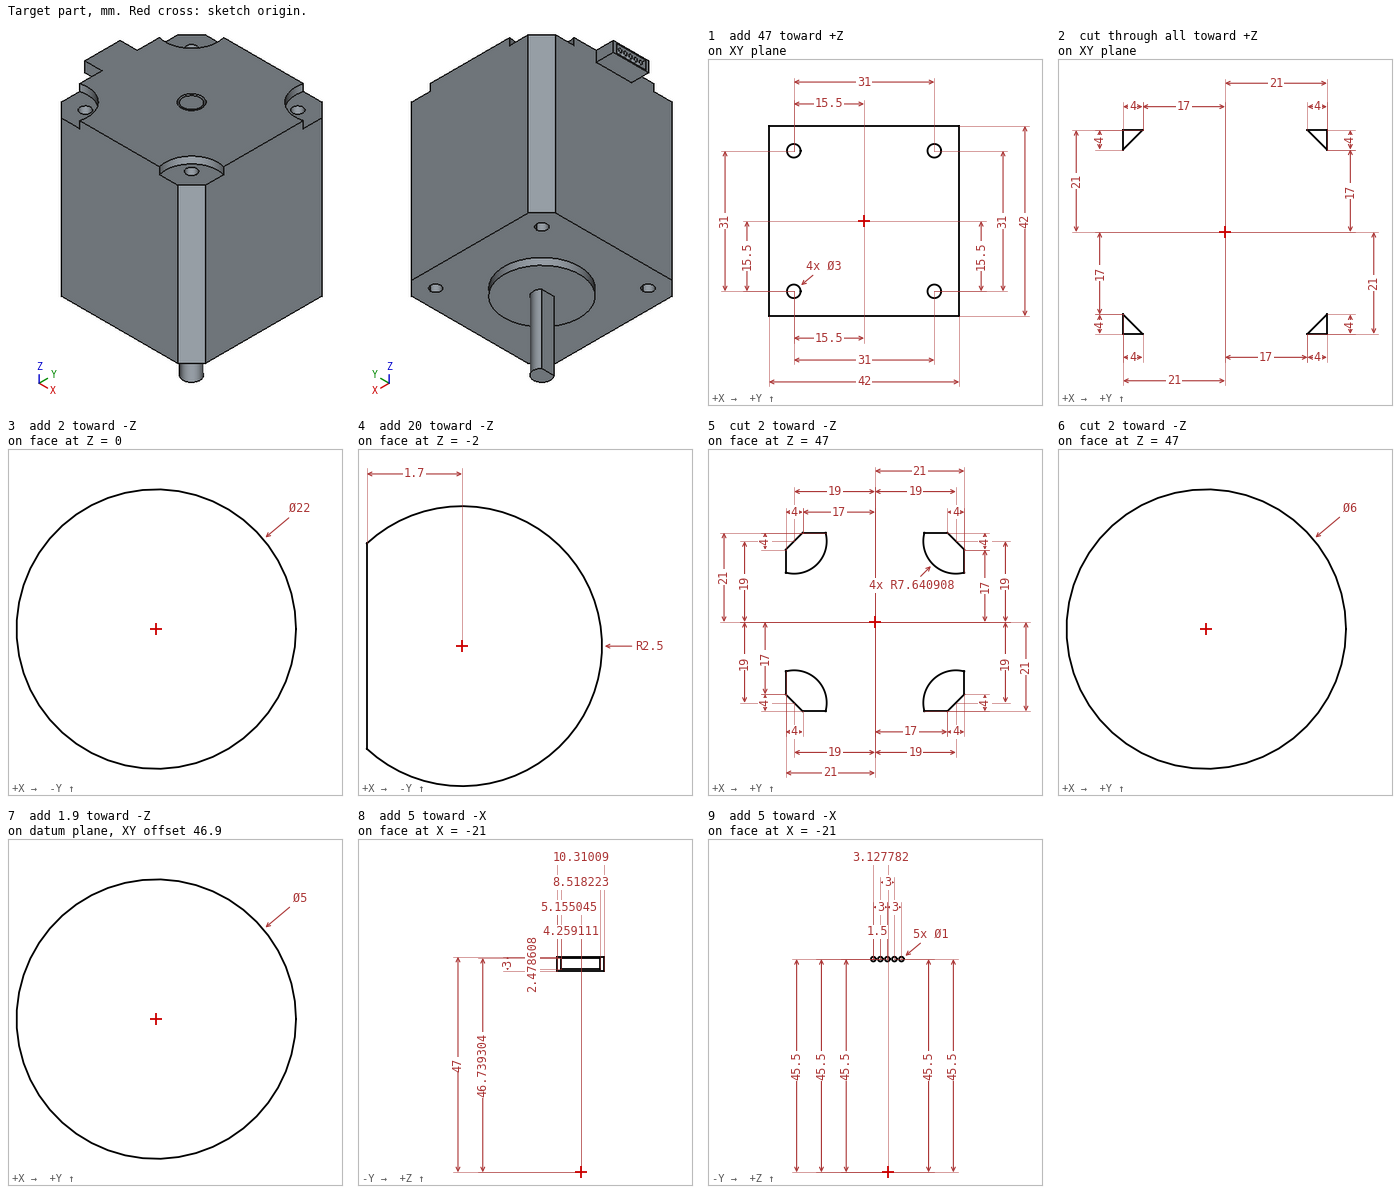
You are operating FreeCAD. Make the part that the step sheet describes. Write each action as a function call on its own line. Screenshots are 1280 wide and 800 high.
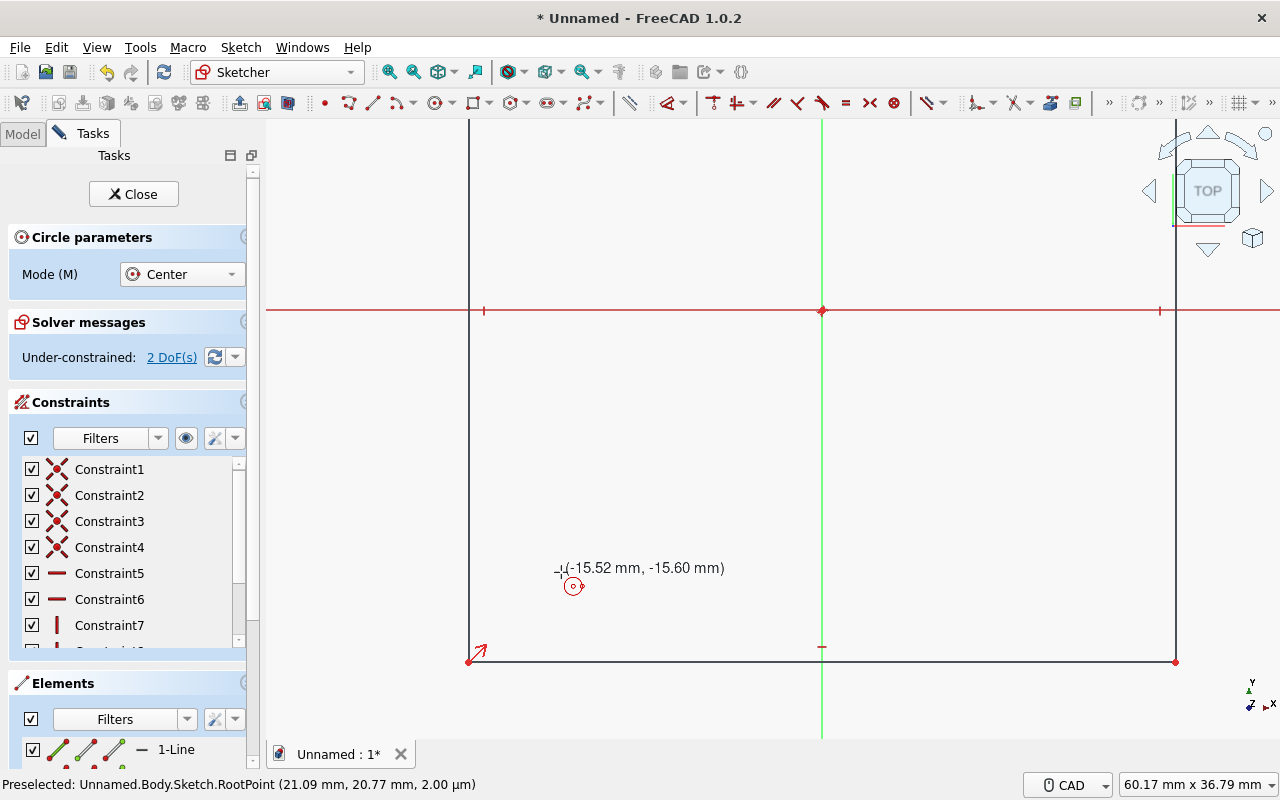
click(561, 572)
click(579, 554)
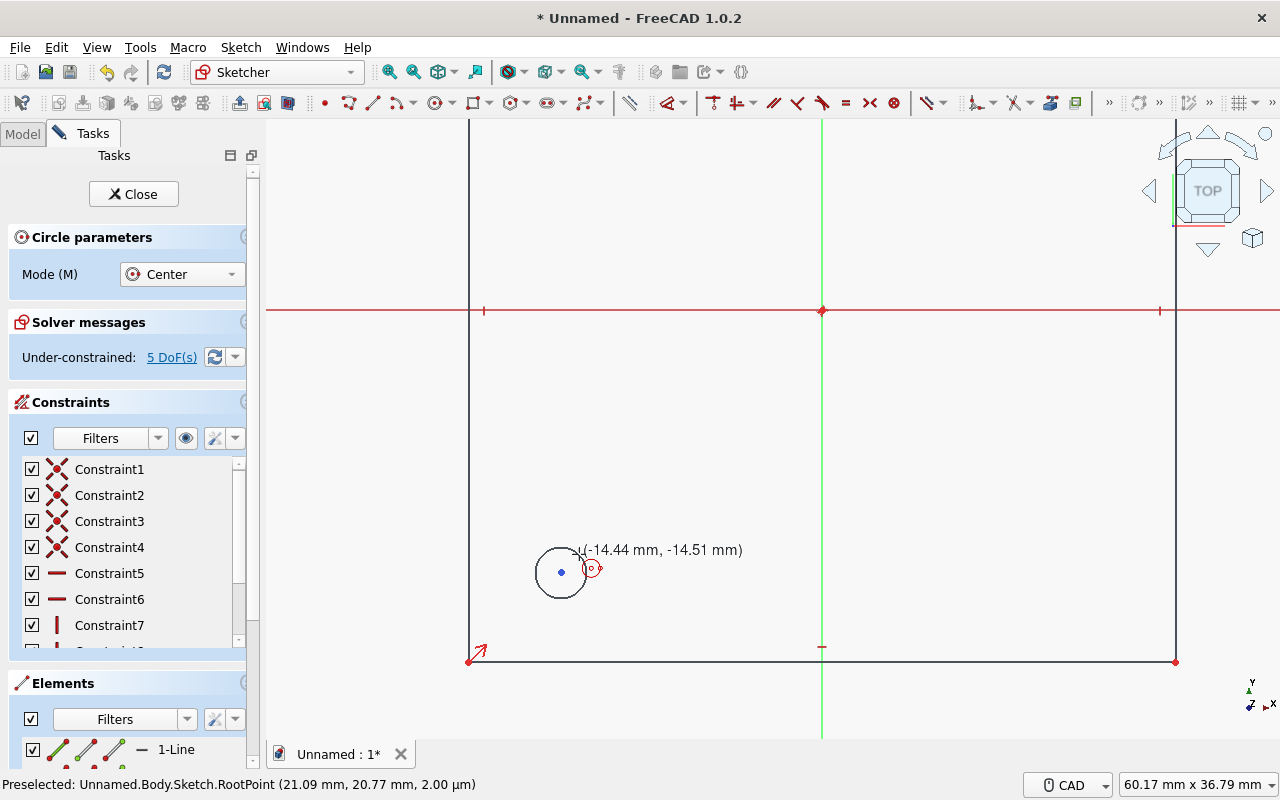
click(1084, 572)
click(1101, 554)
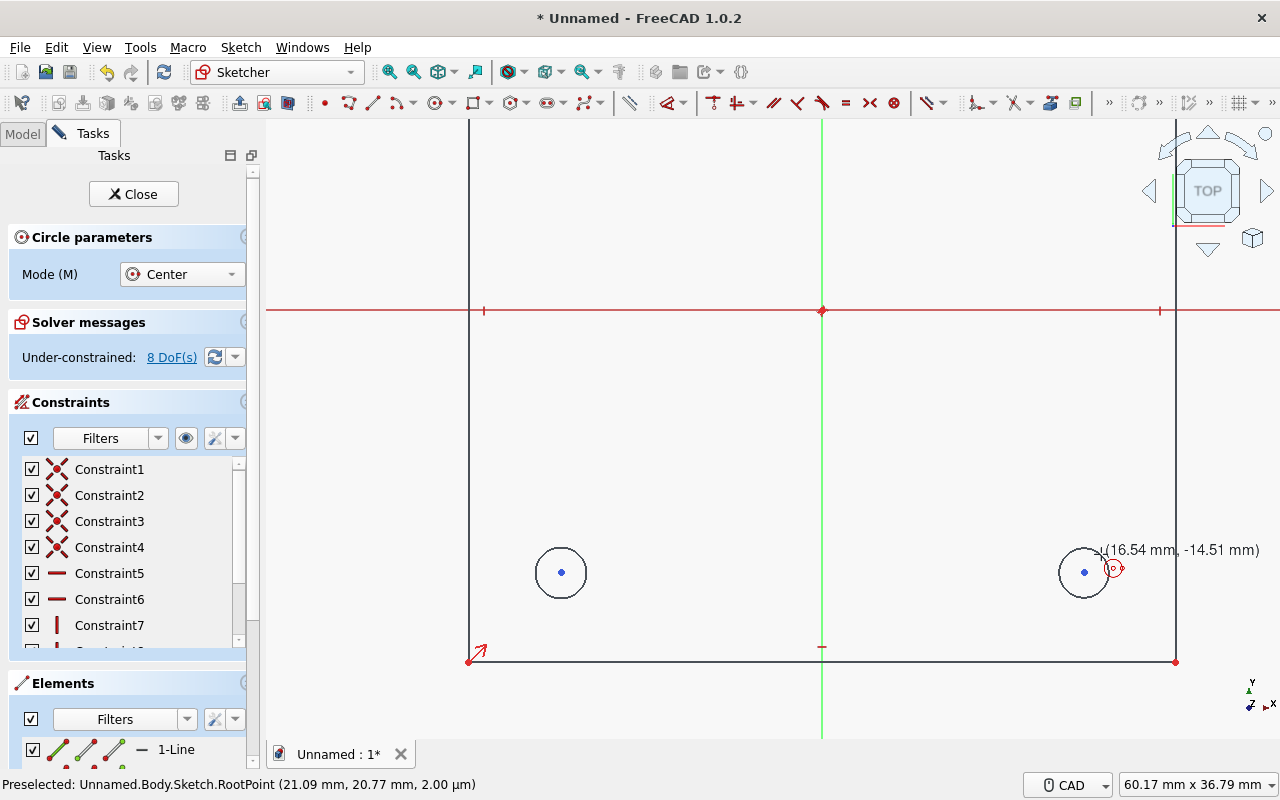
scroll(561, 573, down, 3)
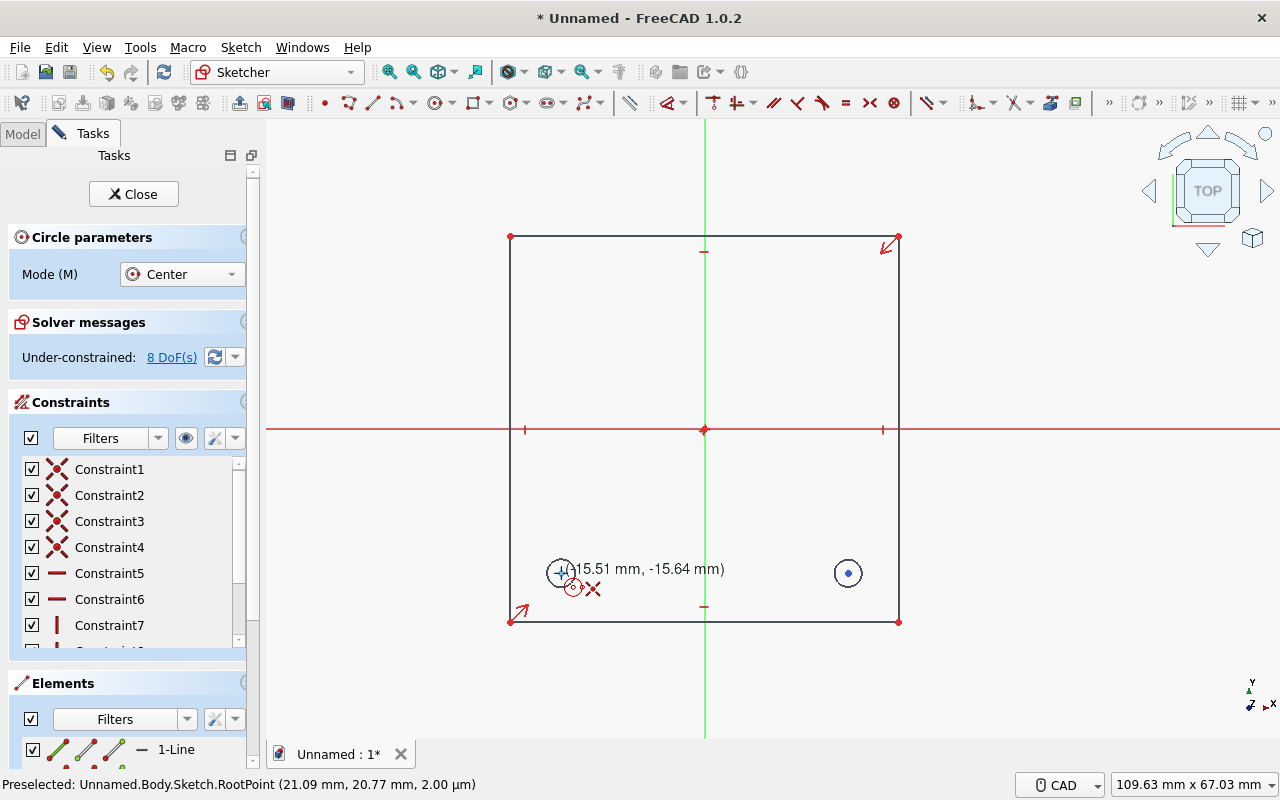
scroll(561, 286, up, 3)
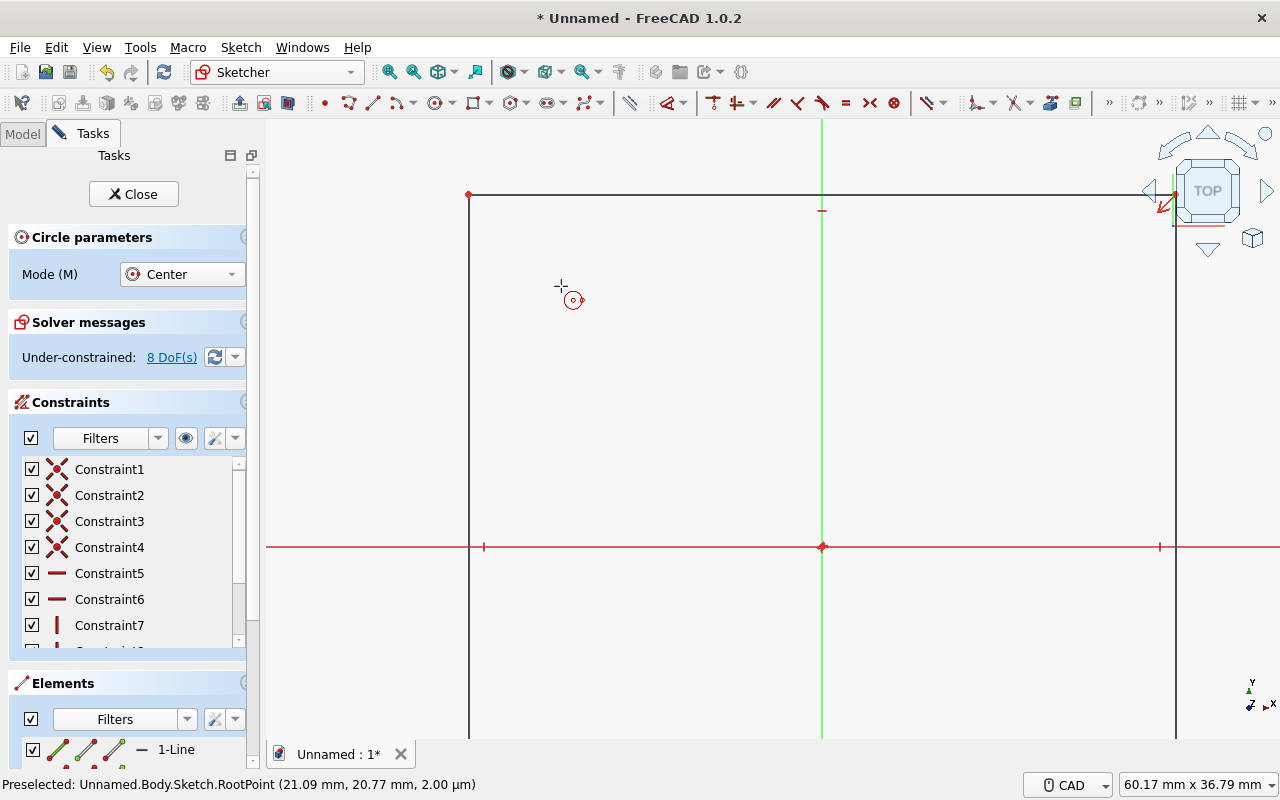
click(561, 285)
click(579, 268)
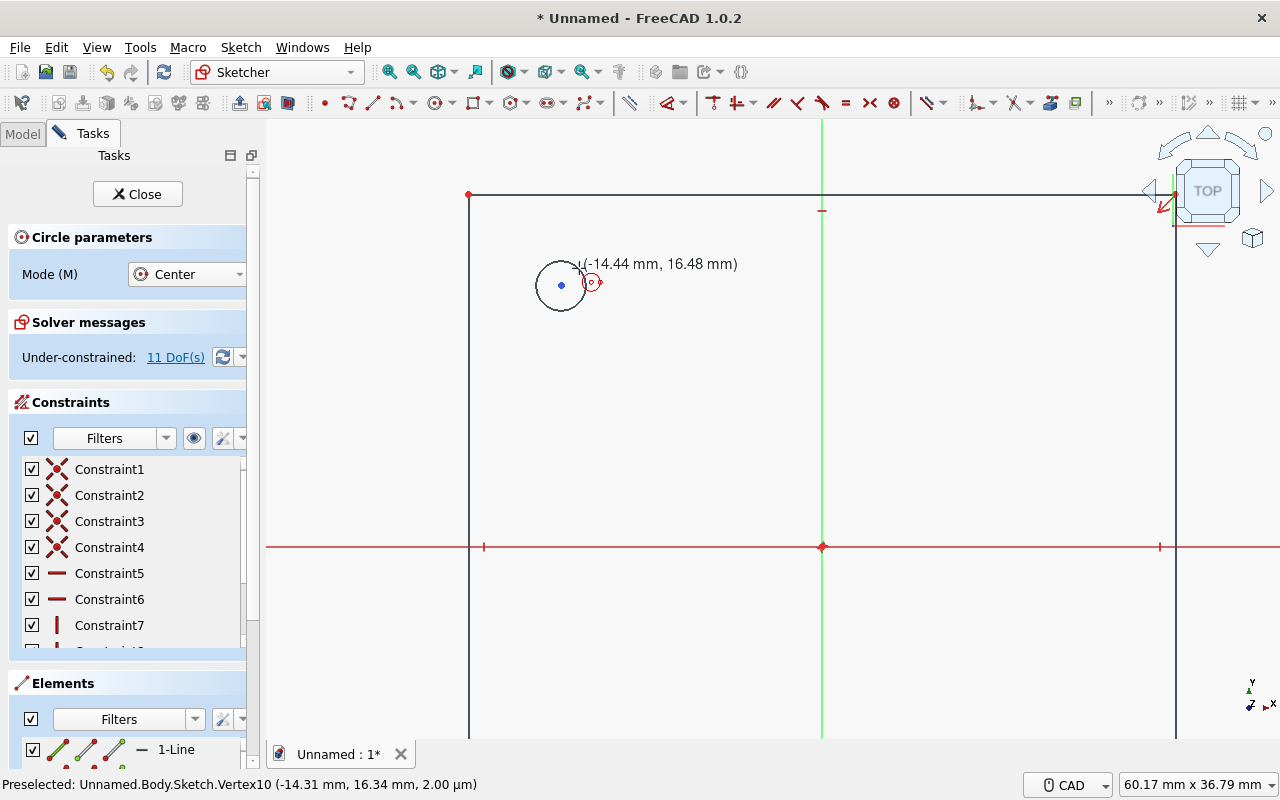
click(1084, 285)
click(1101, 268)
key(Escape)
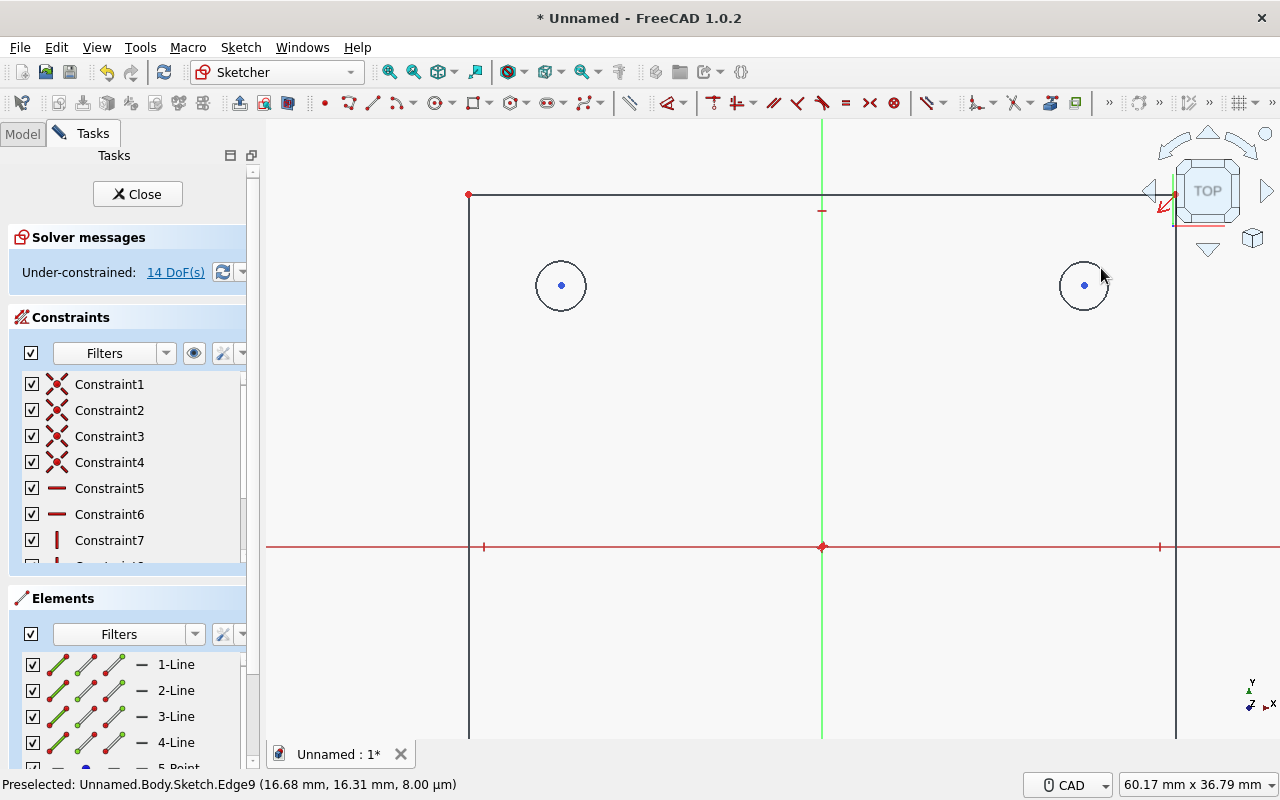
scroll(561, 286, down, 3)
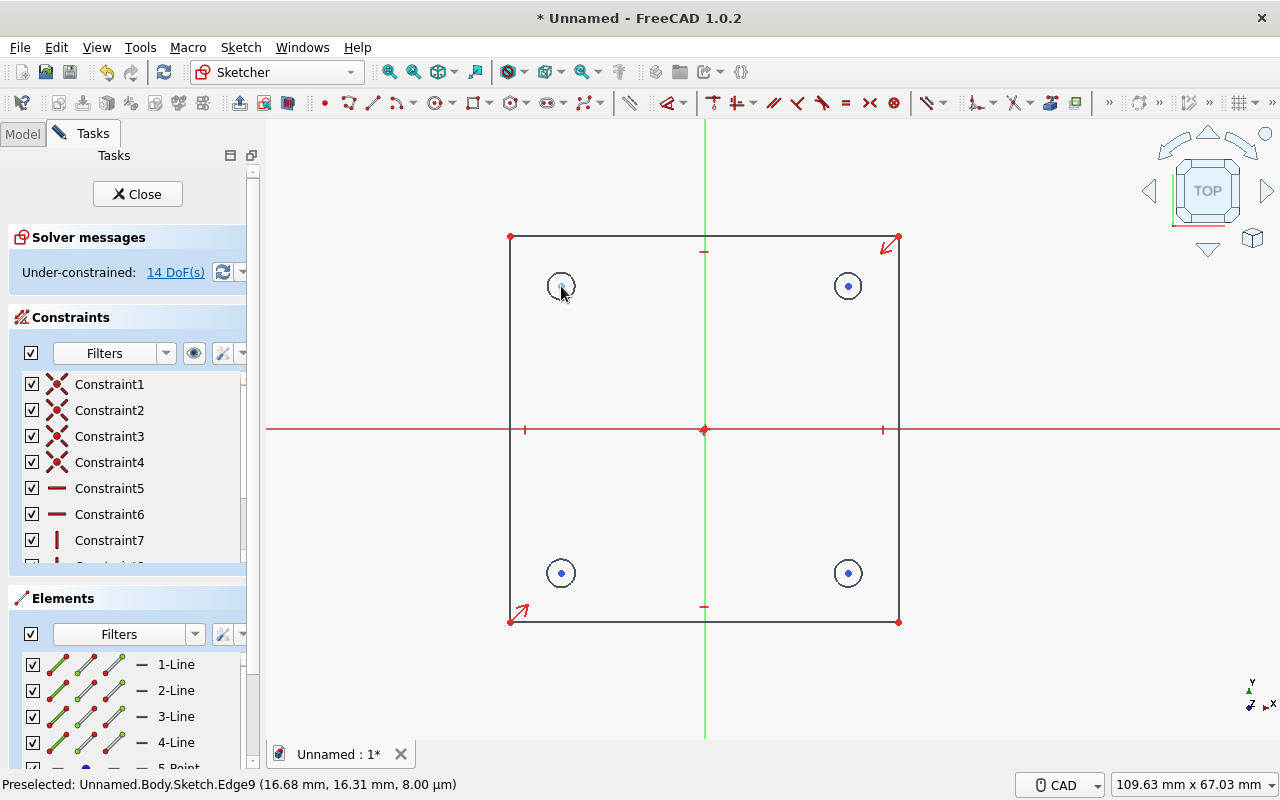
click(571, 563)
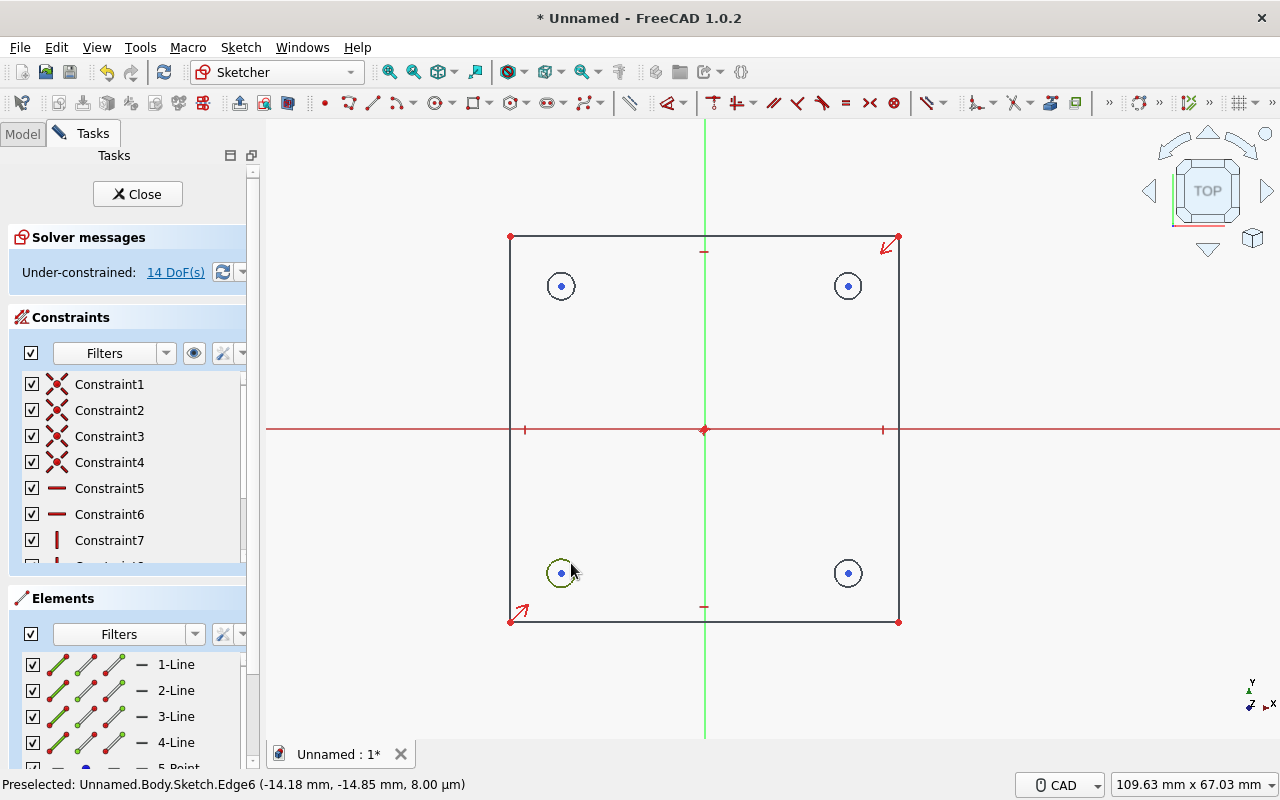
click(858, 564)